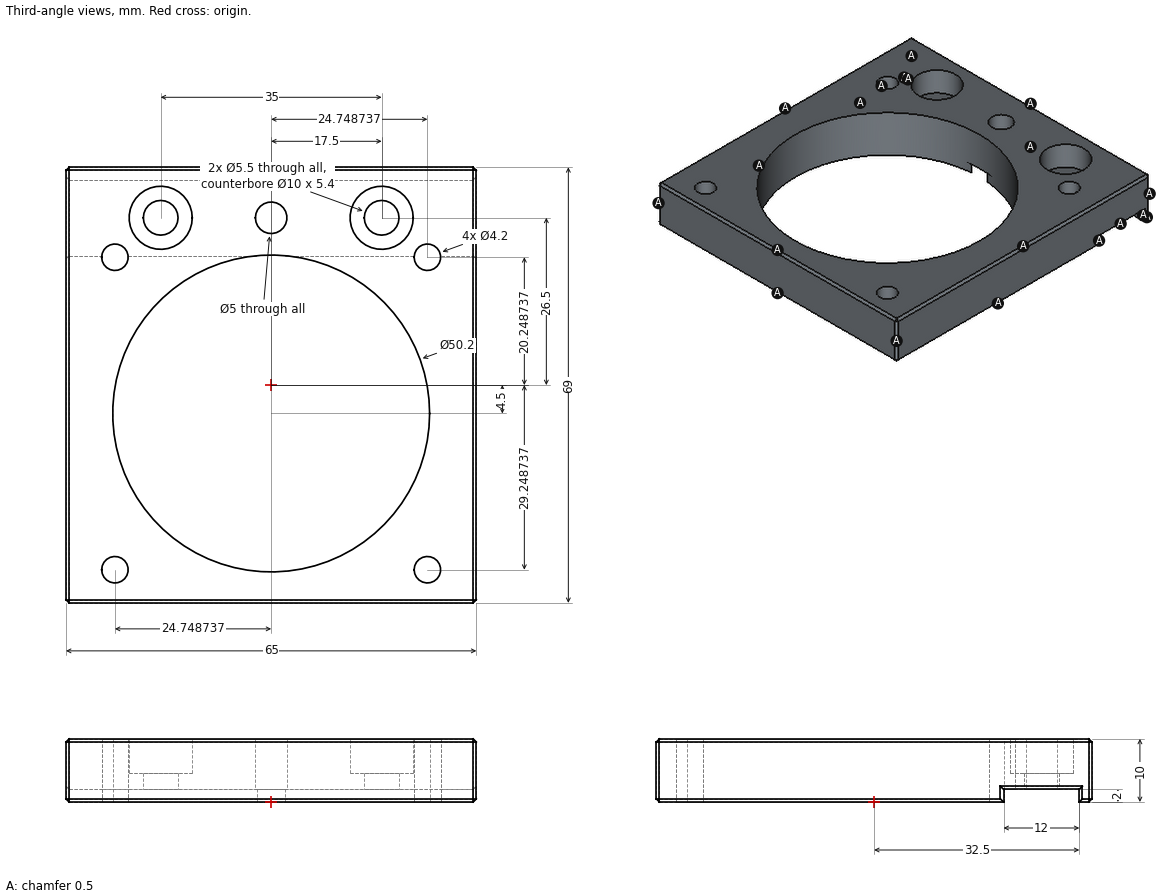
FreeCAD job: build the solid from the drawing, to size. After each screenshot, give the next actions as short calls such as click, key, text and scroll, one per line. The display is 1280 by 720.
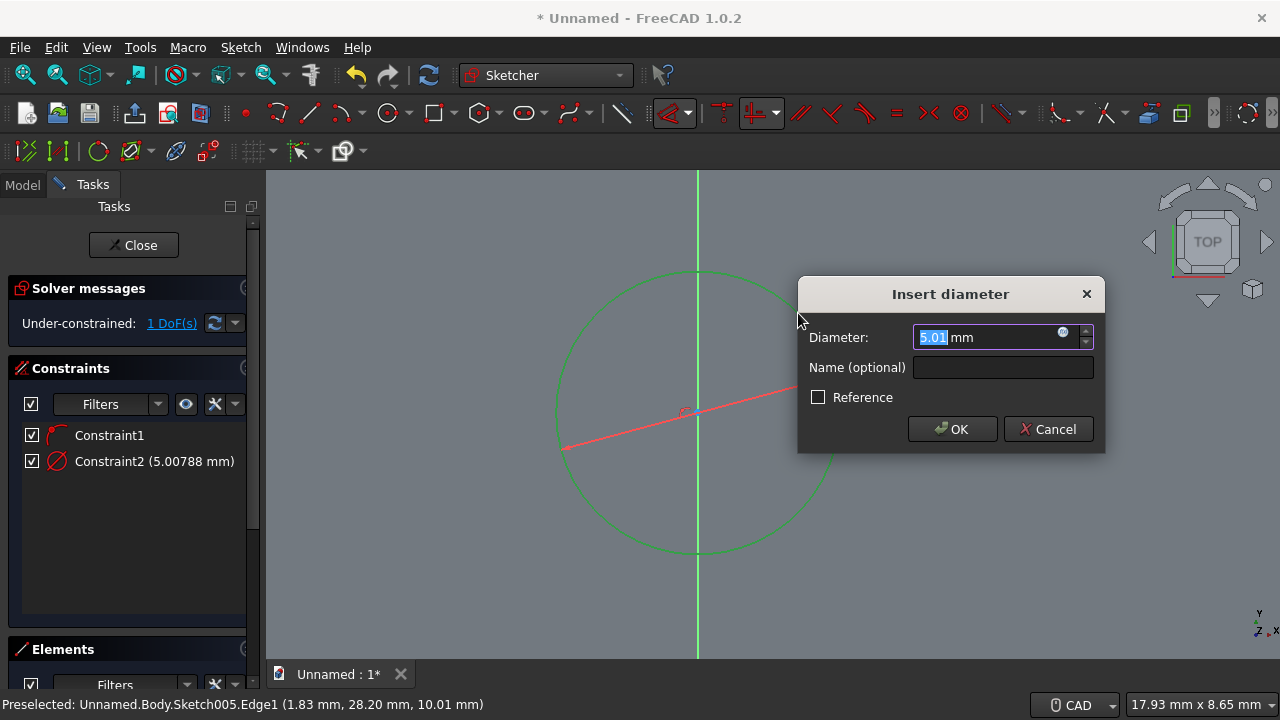
text(5)
key(Return)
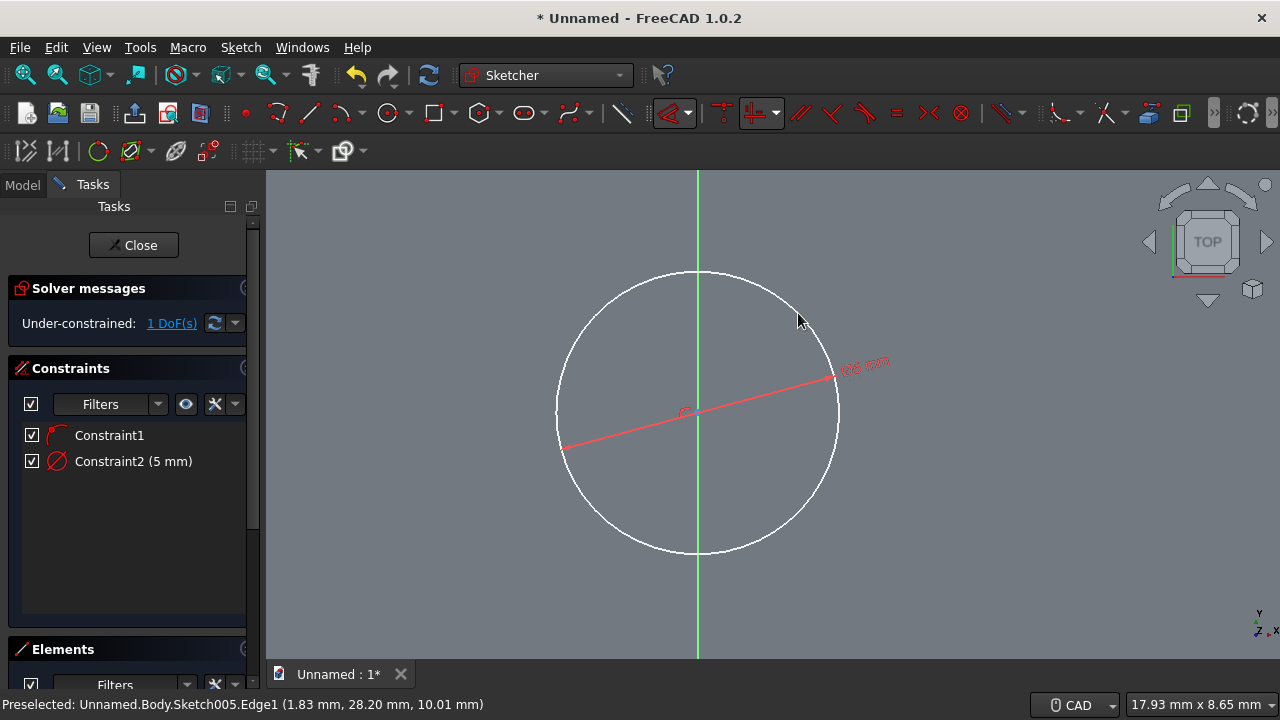
click(698, 413)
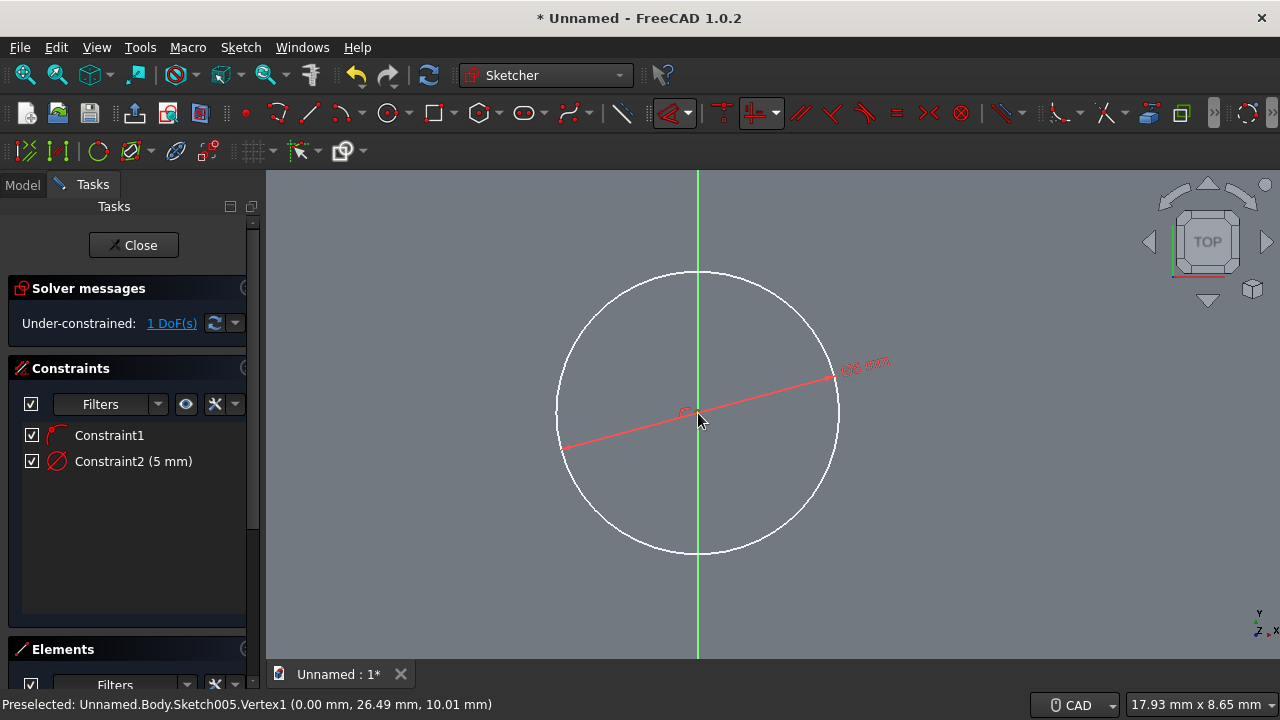
key(i)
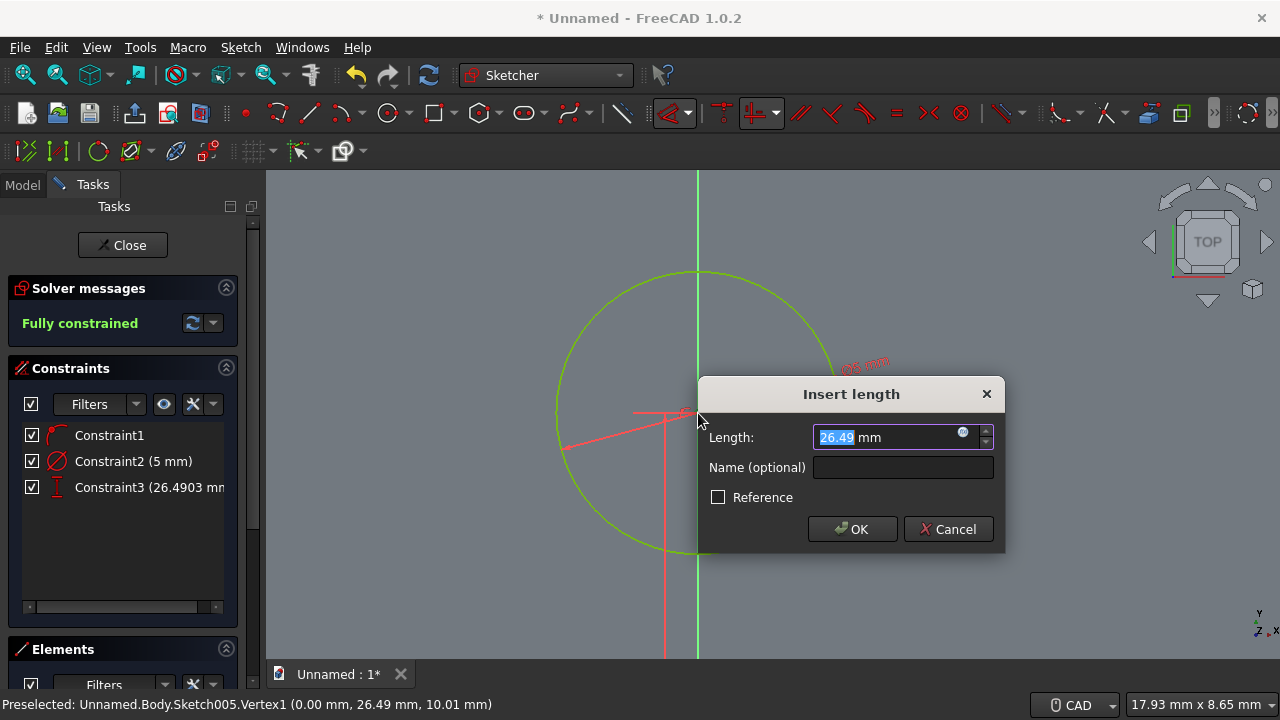
text(26.5)
key(Return)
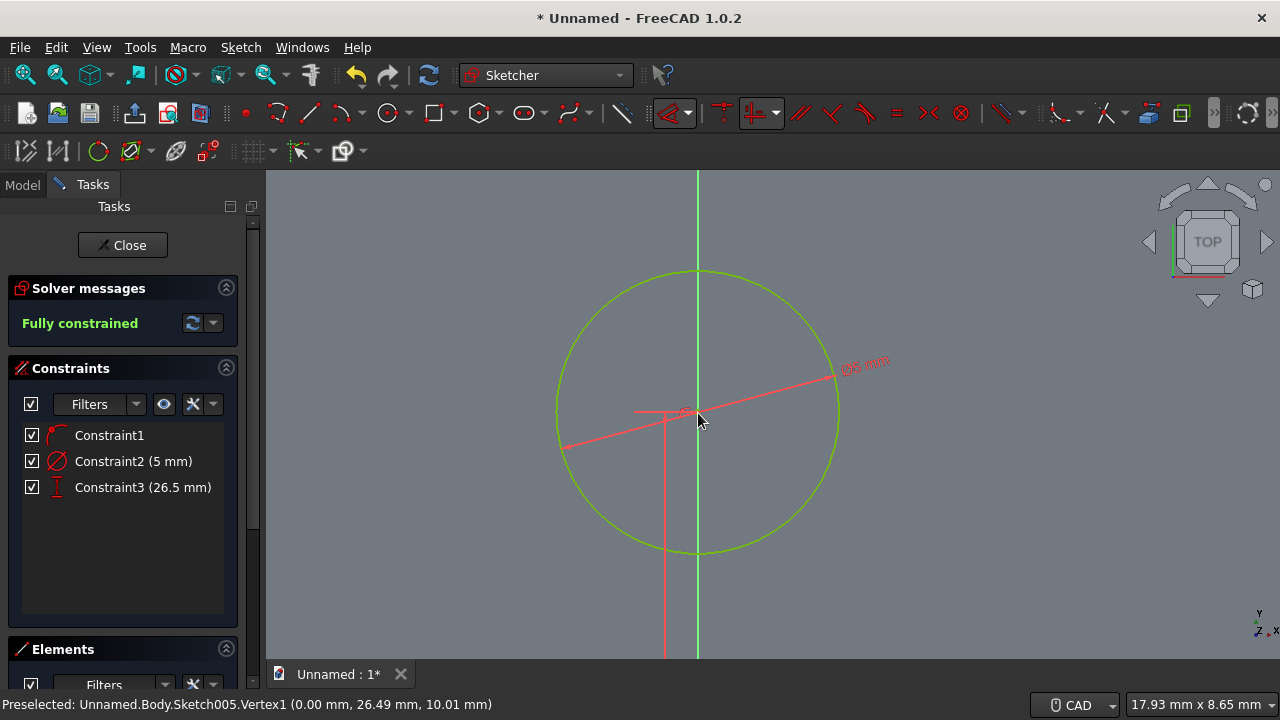
click(123, 245)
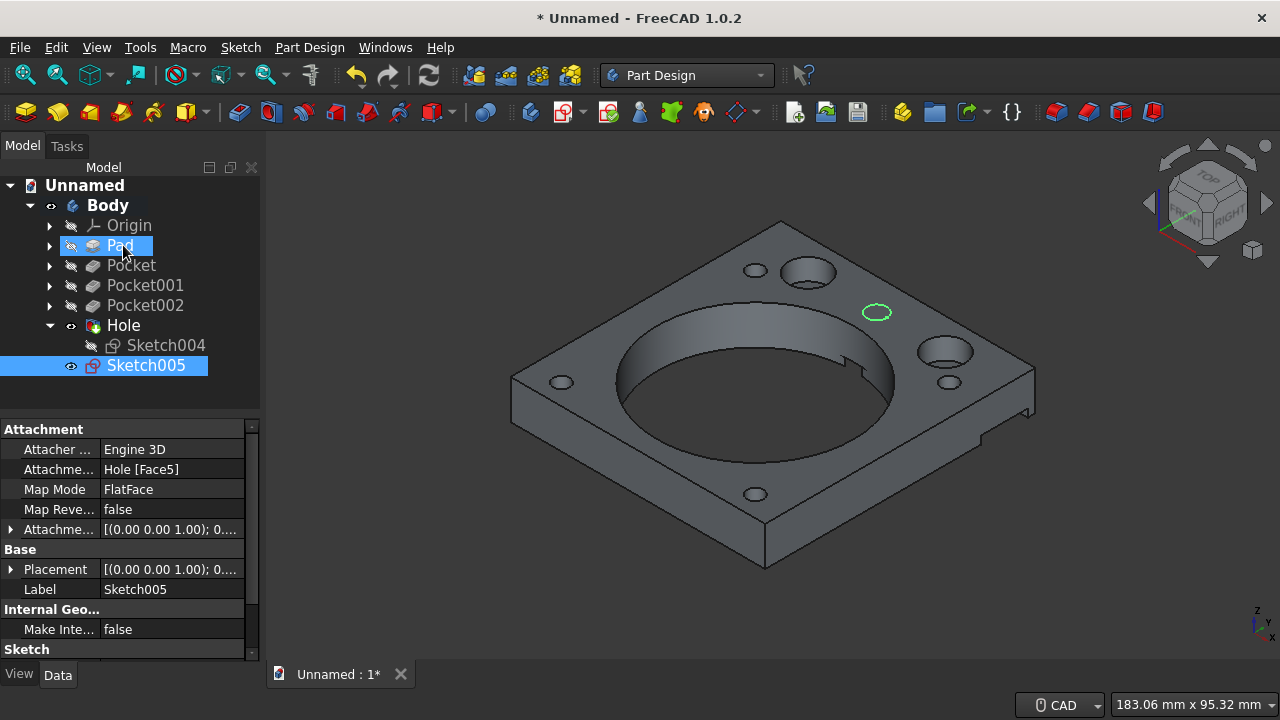
click(272, 112)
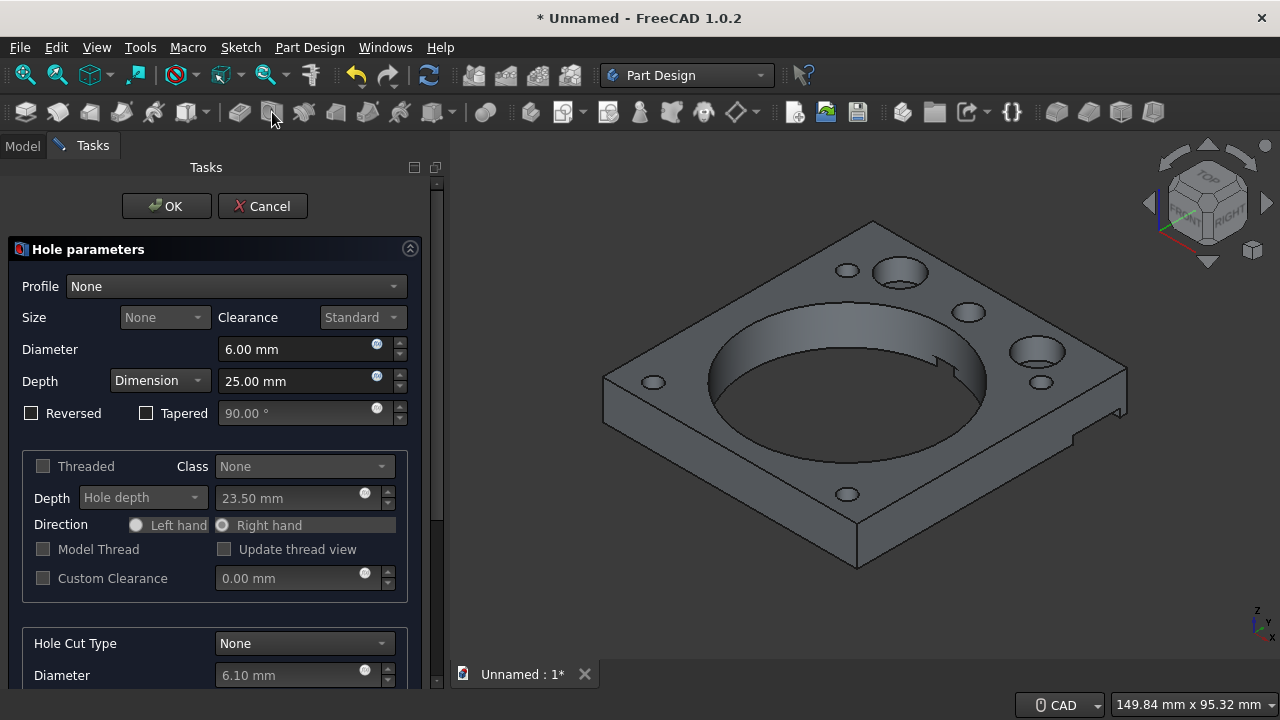
triple_click(305, 349)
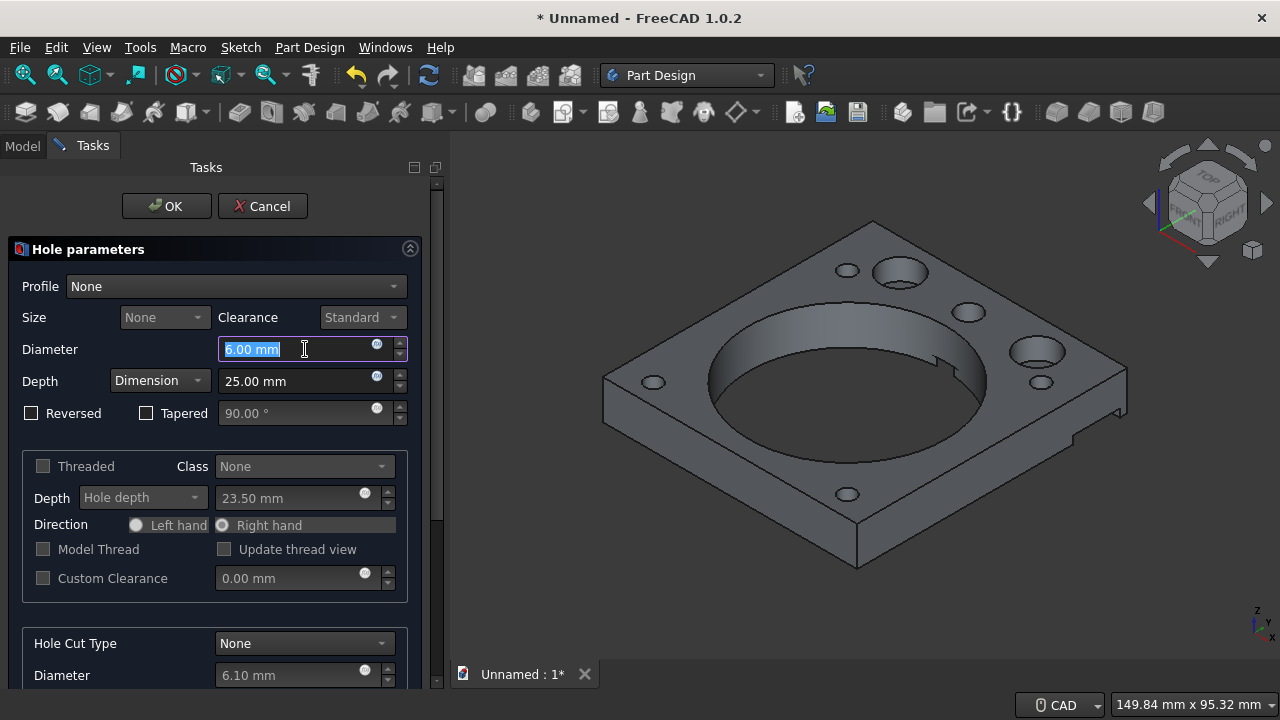
text(5)
key(Tab)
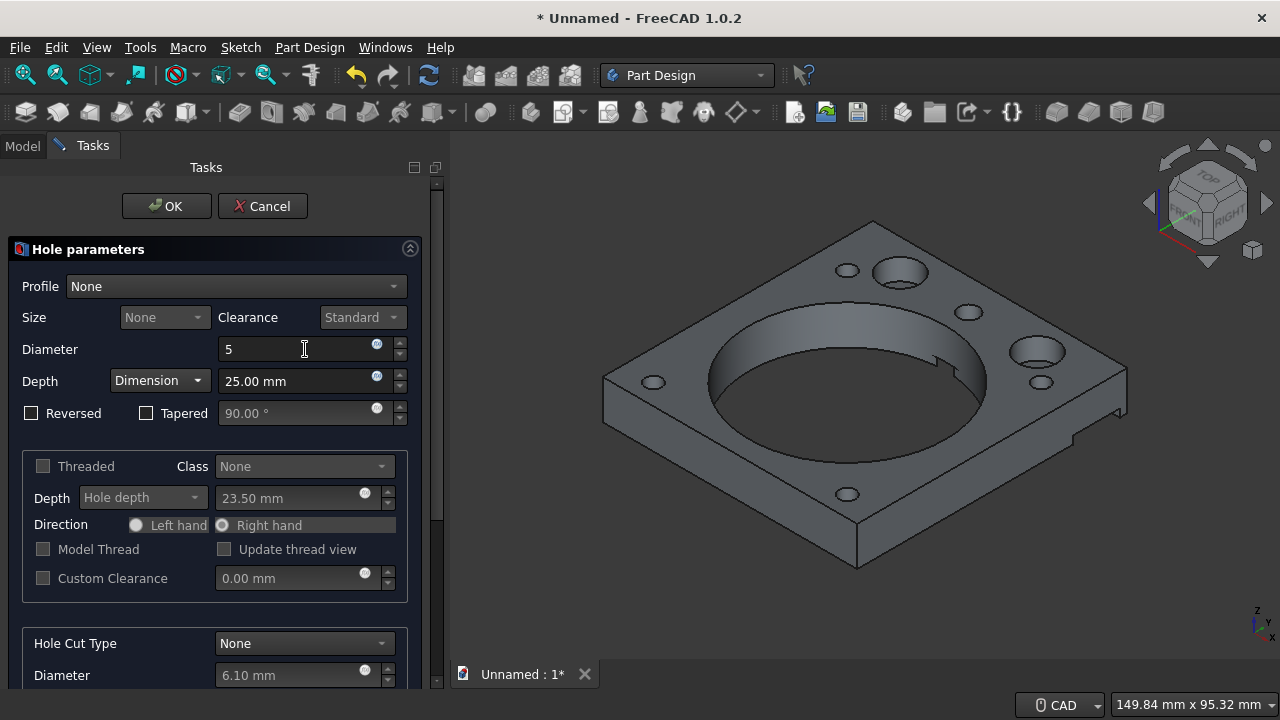
click(161, 380)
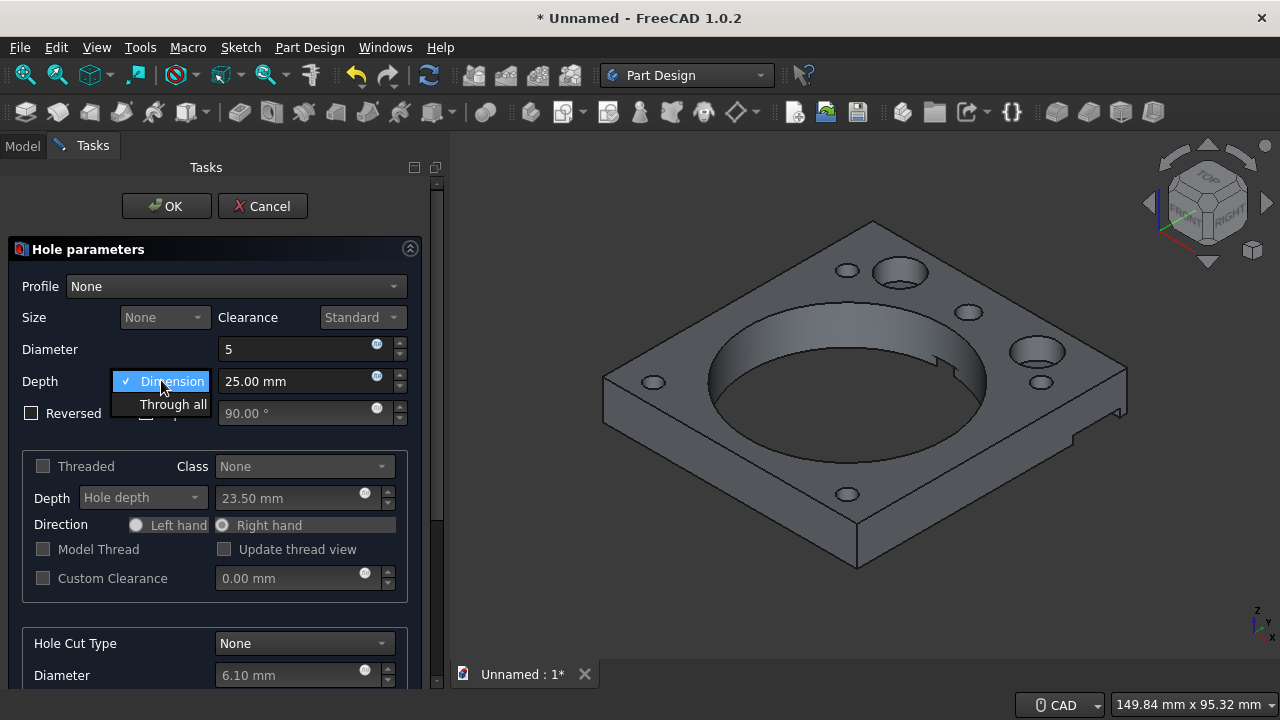
click(160, 404)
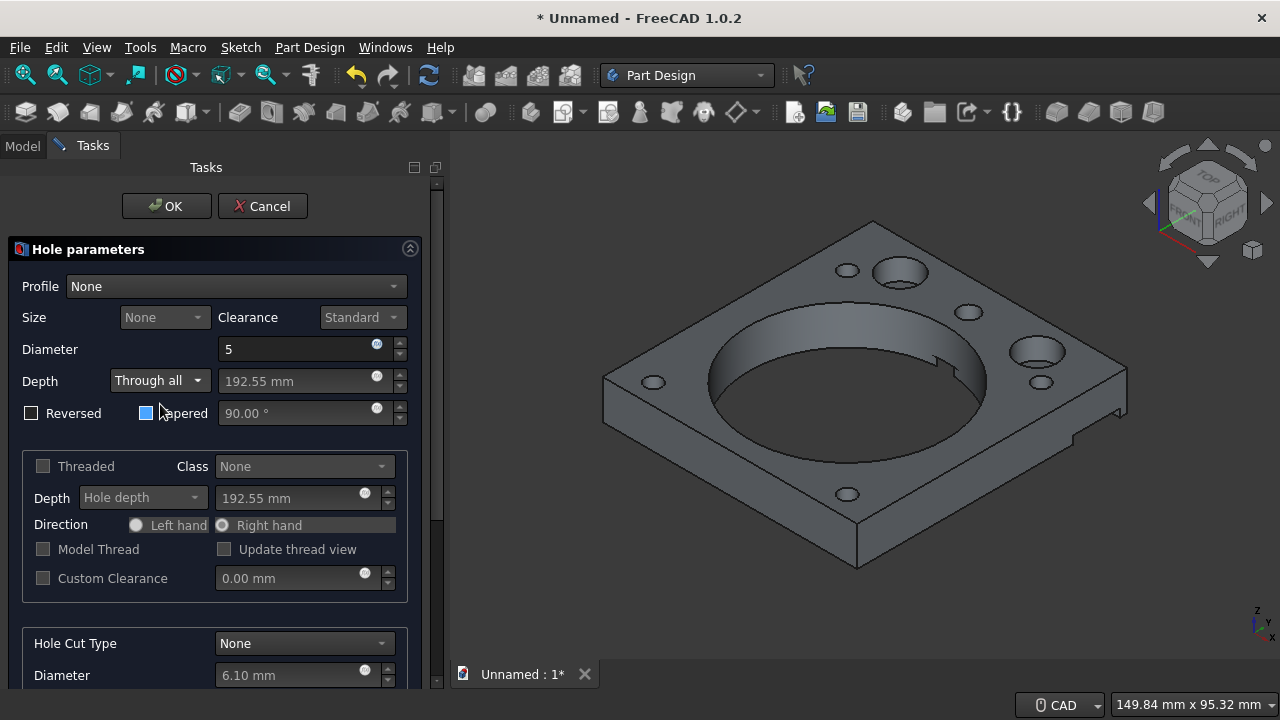
click(167, 206)